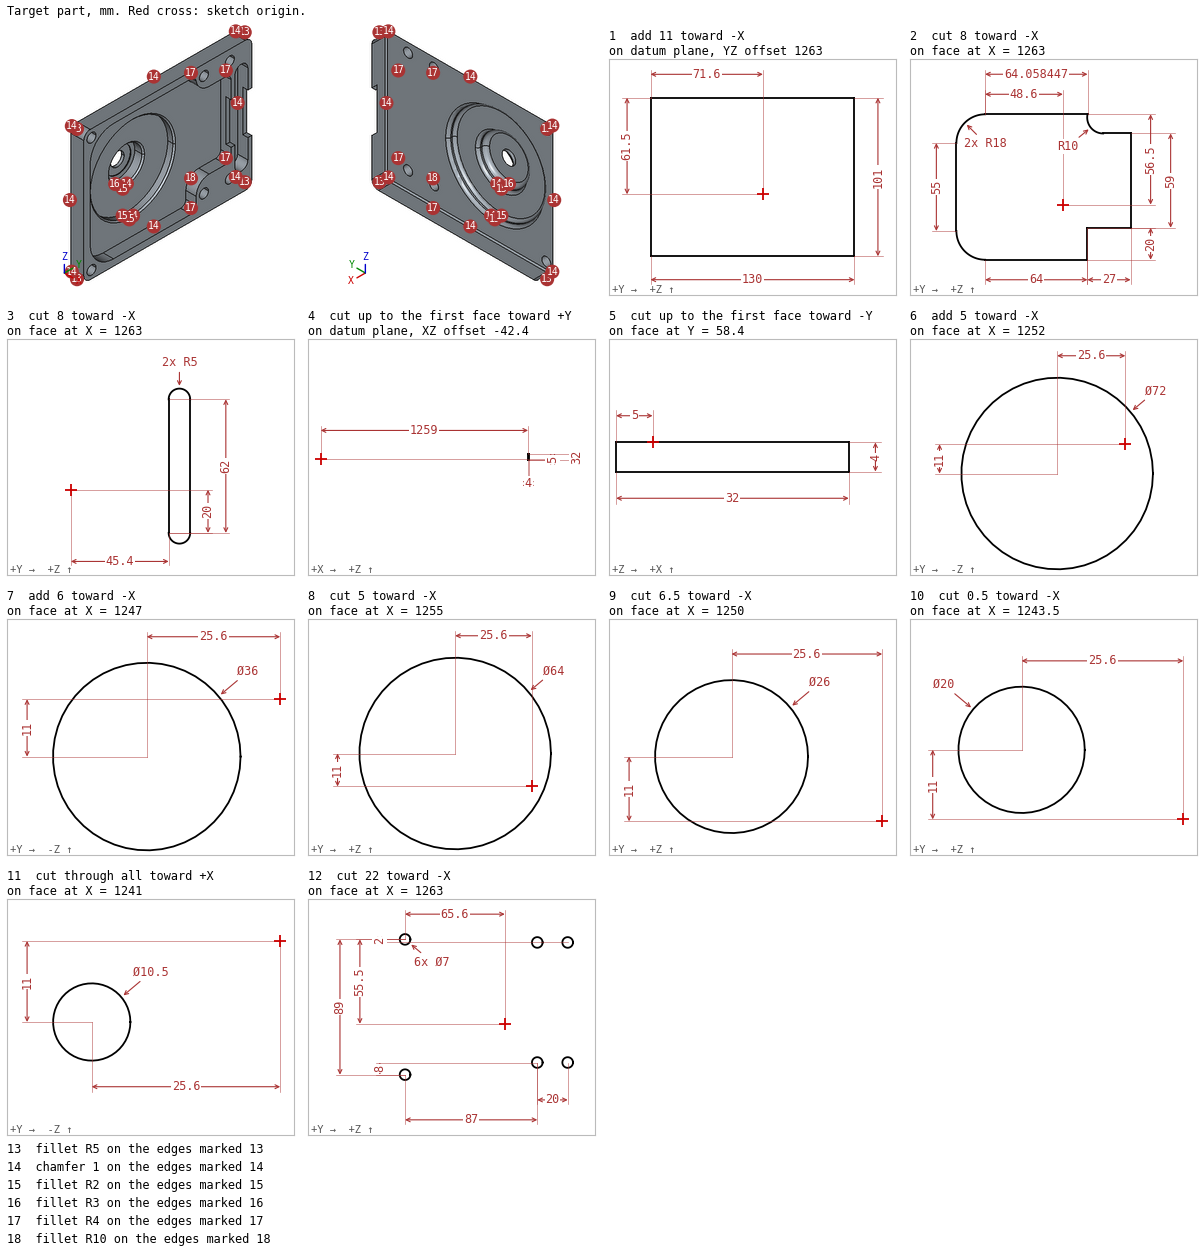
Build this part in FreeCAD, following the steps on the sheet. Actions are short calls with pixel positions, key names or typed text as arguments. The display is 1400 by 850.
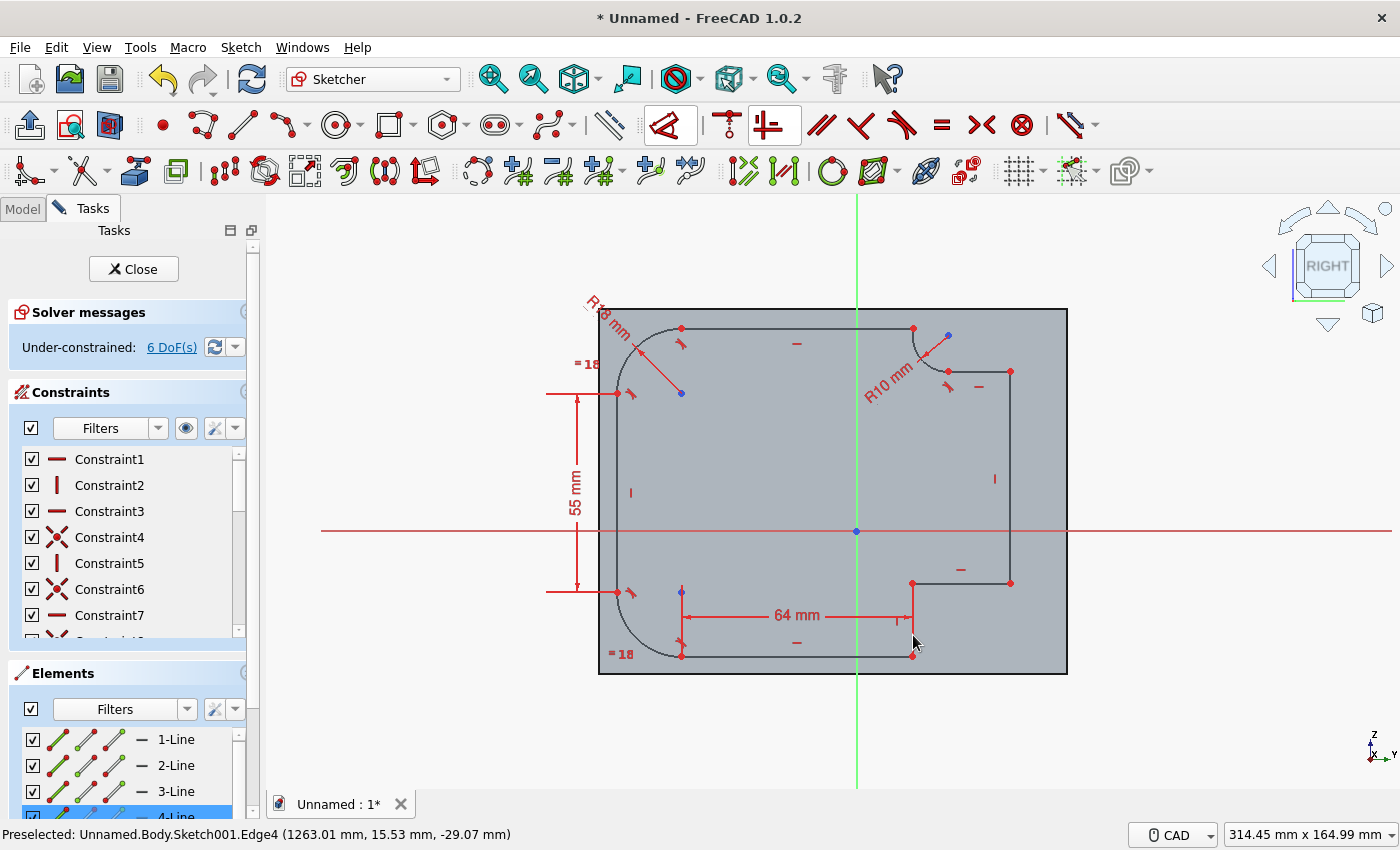
key(i)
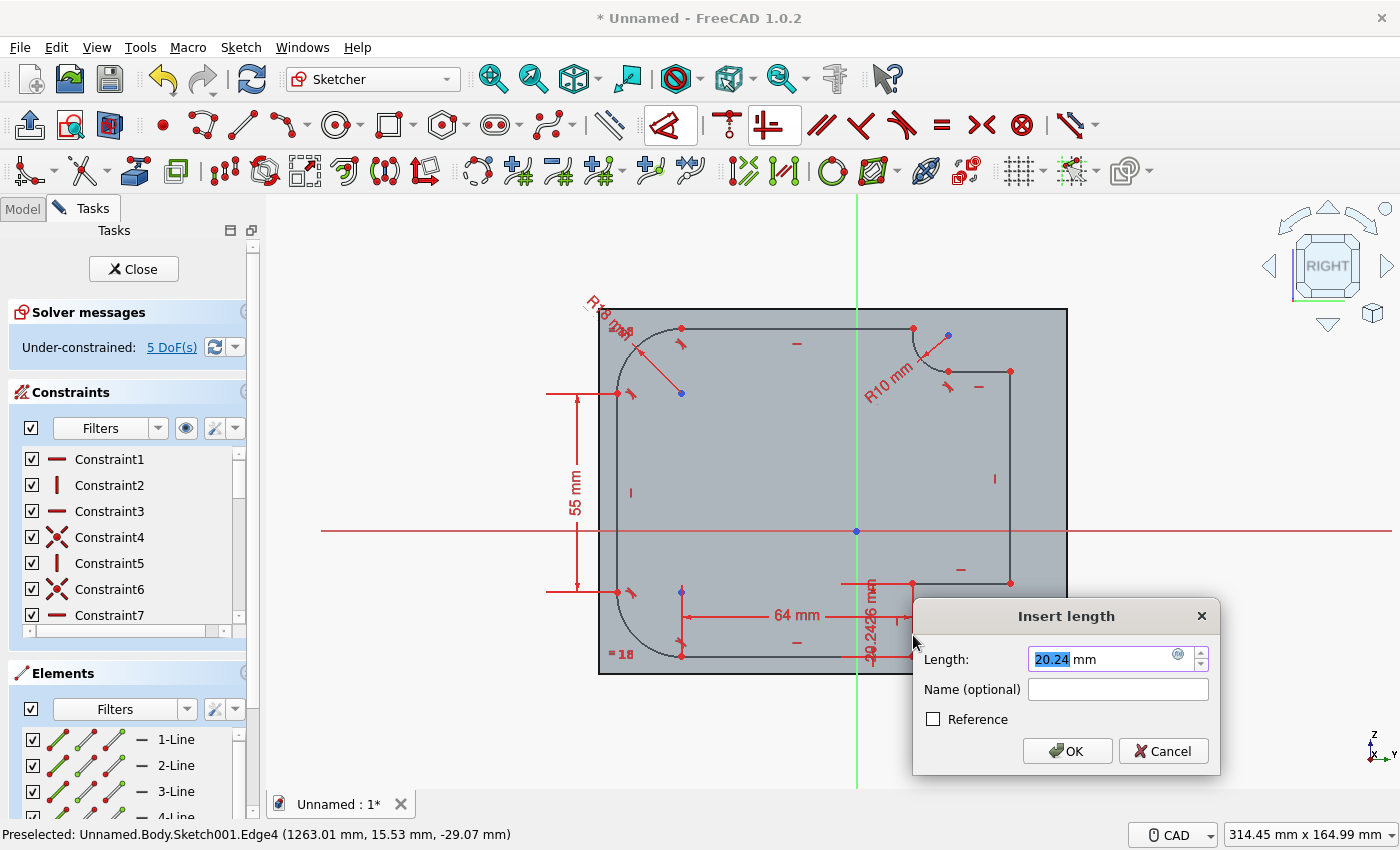
text(20)
key(Return)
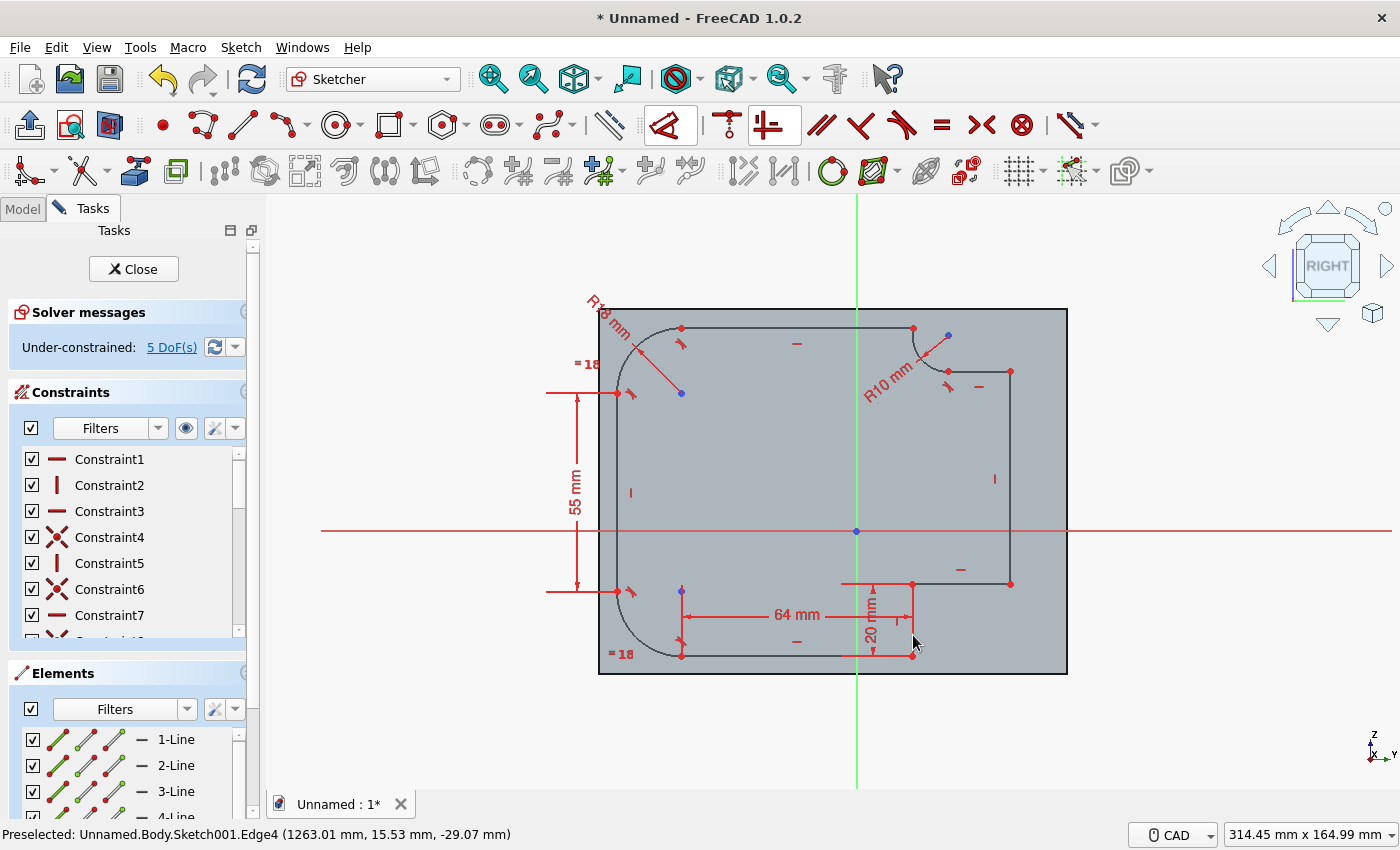
click(942, 584)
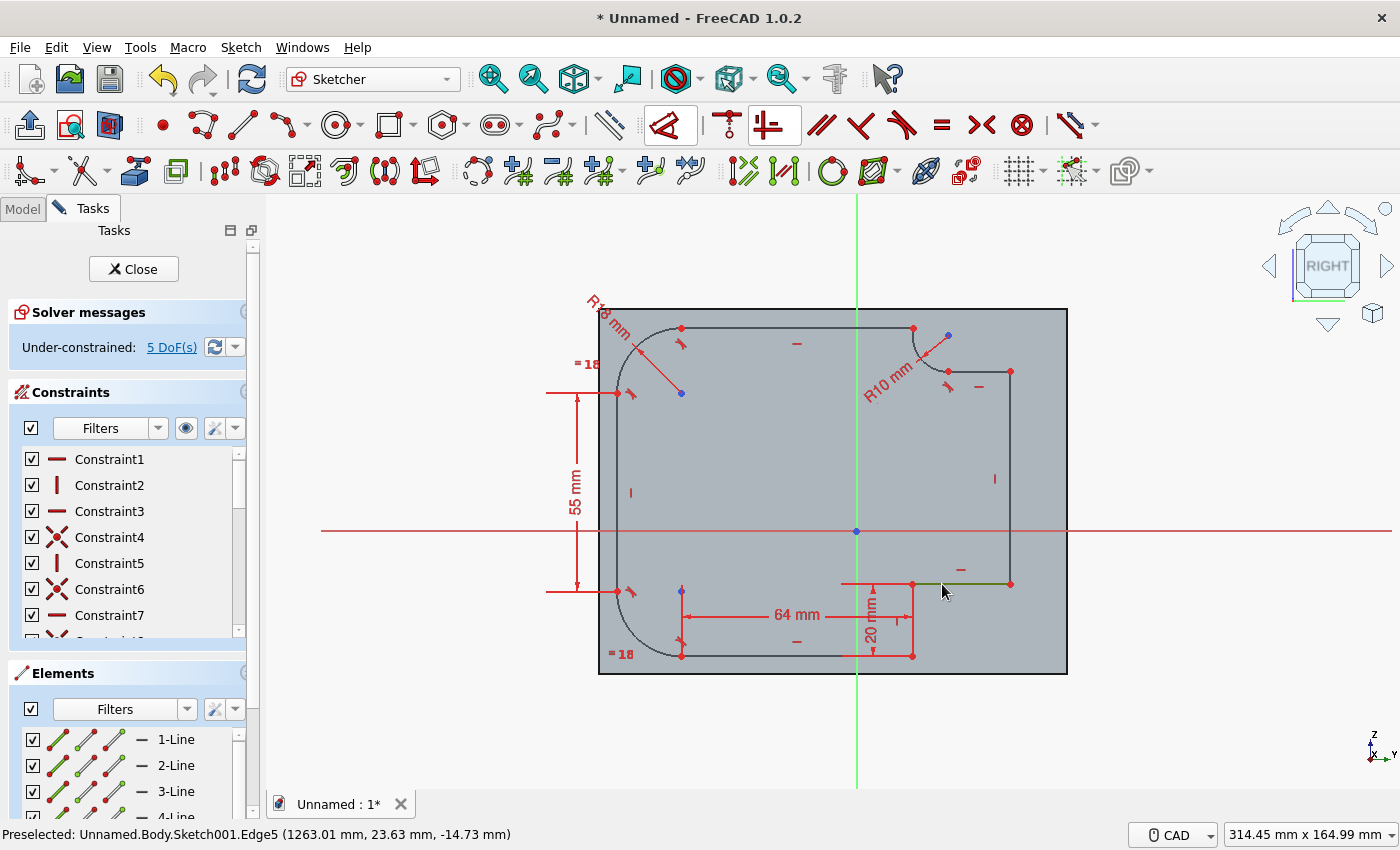
key(l)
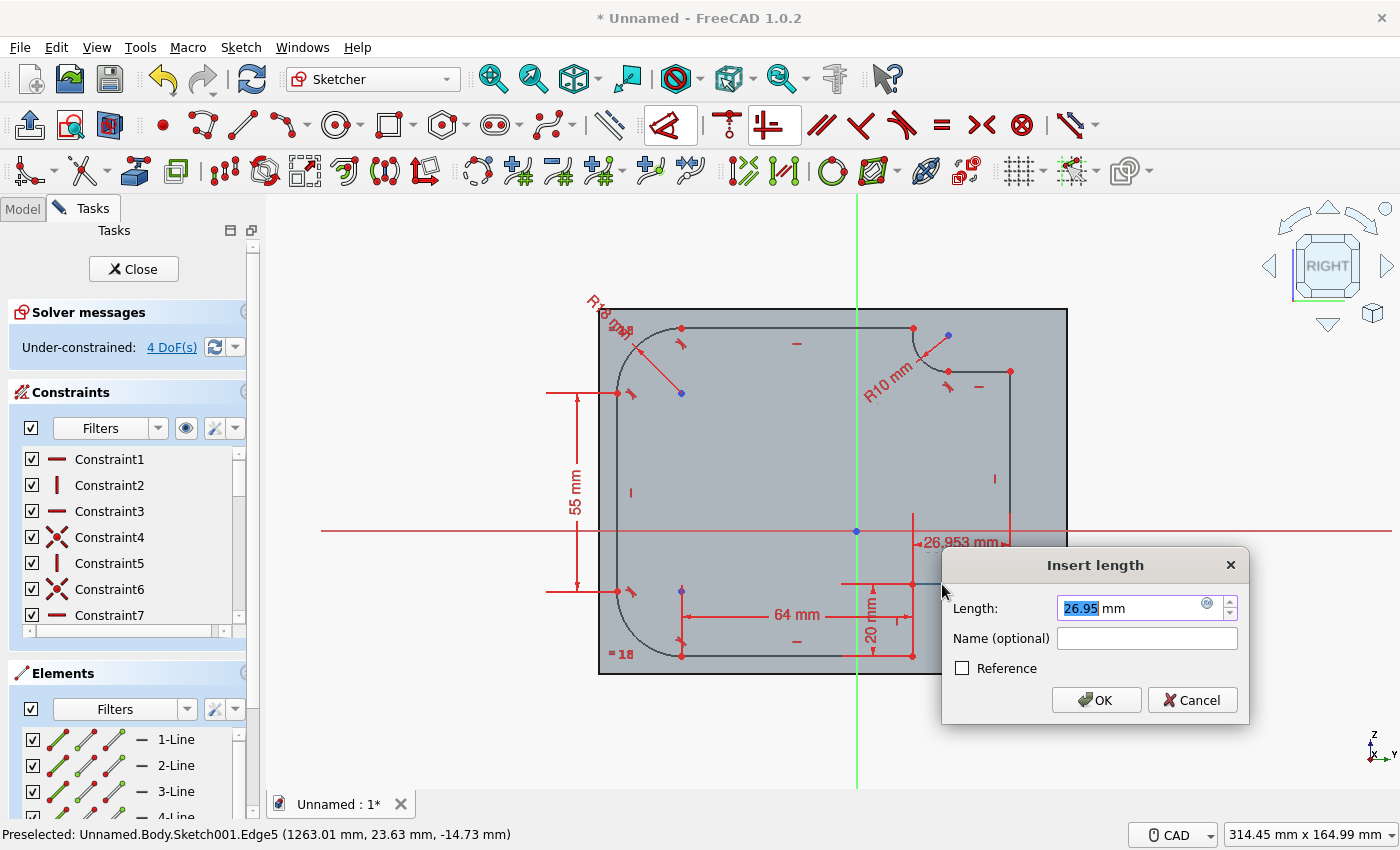
text(27)
key(Return)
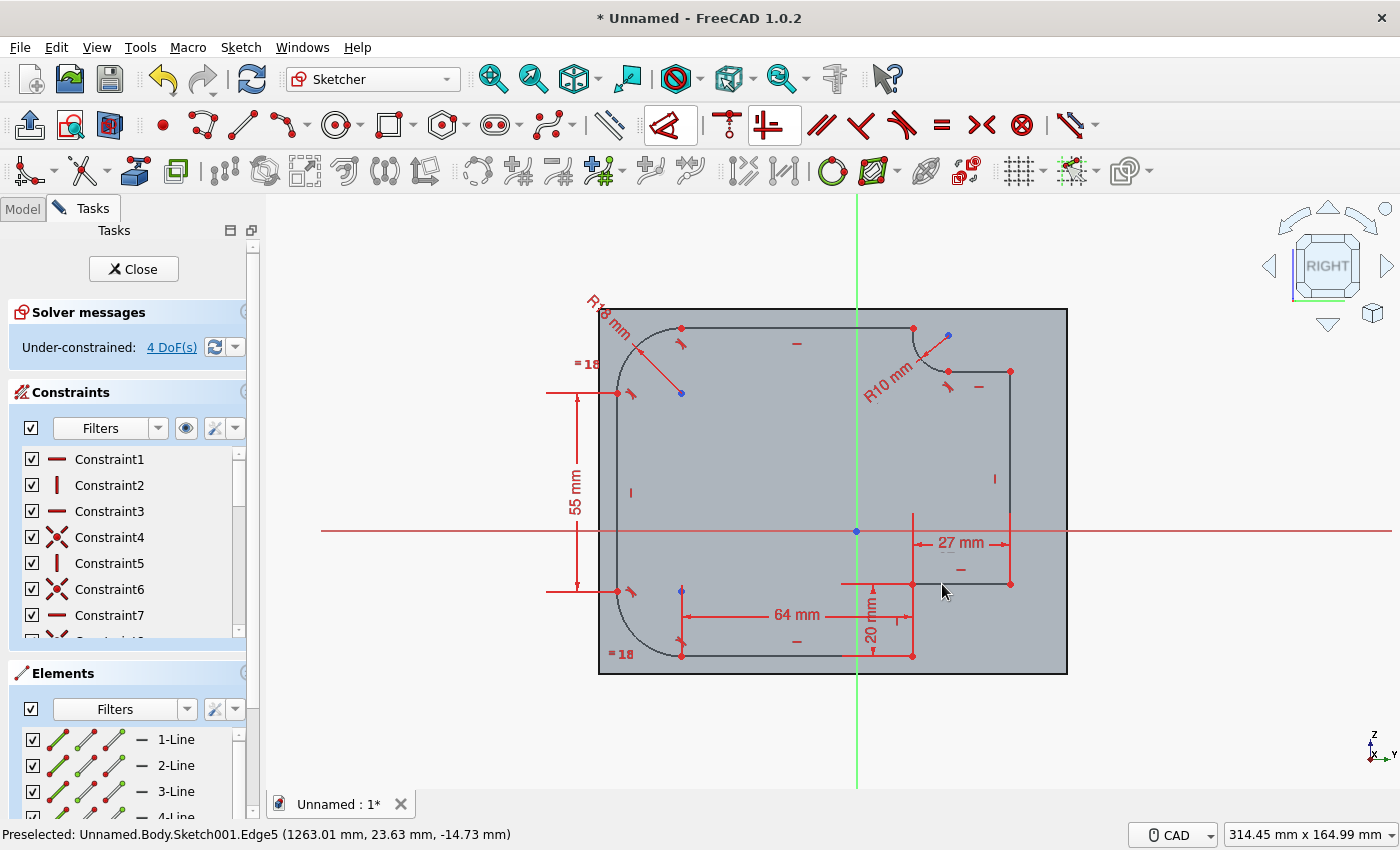
scroll(1010, 521, up, 2)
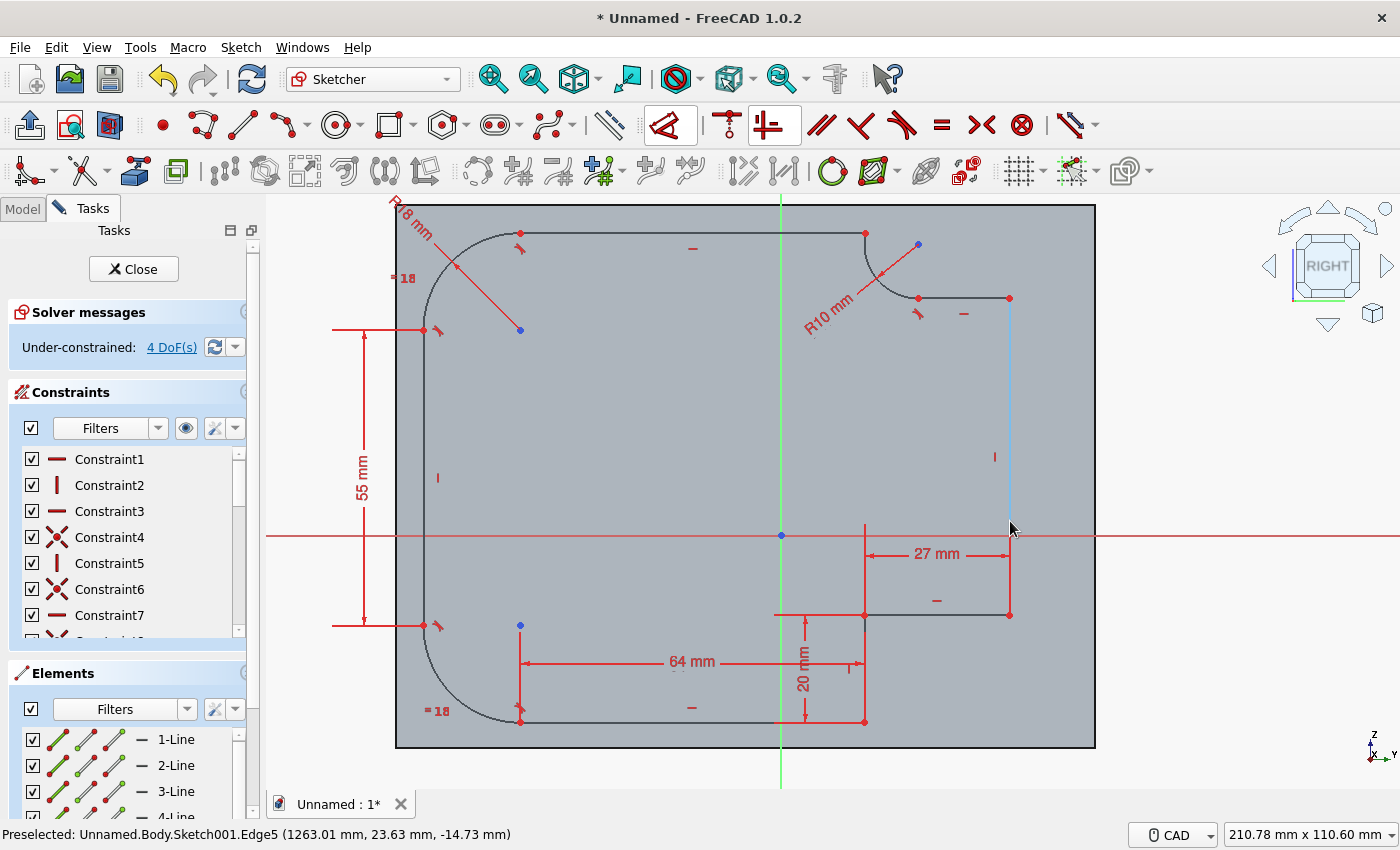
click(1010, 520)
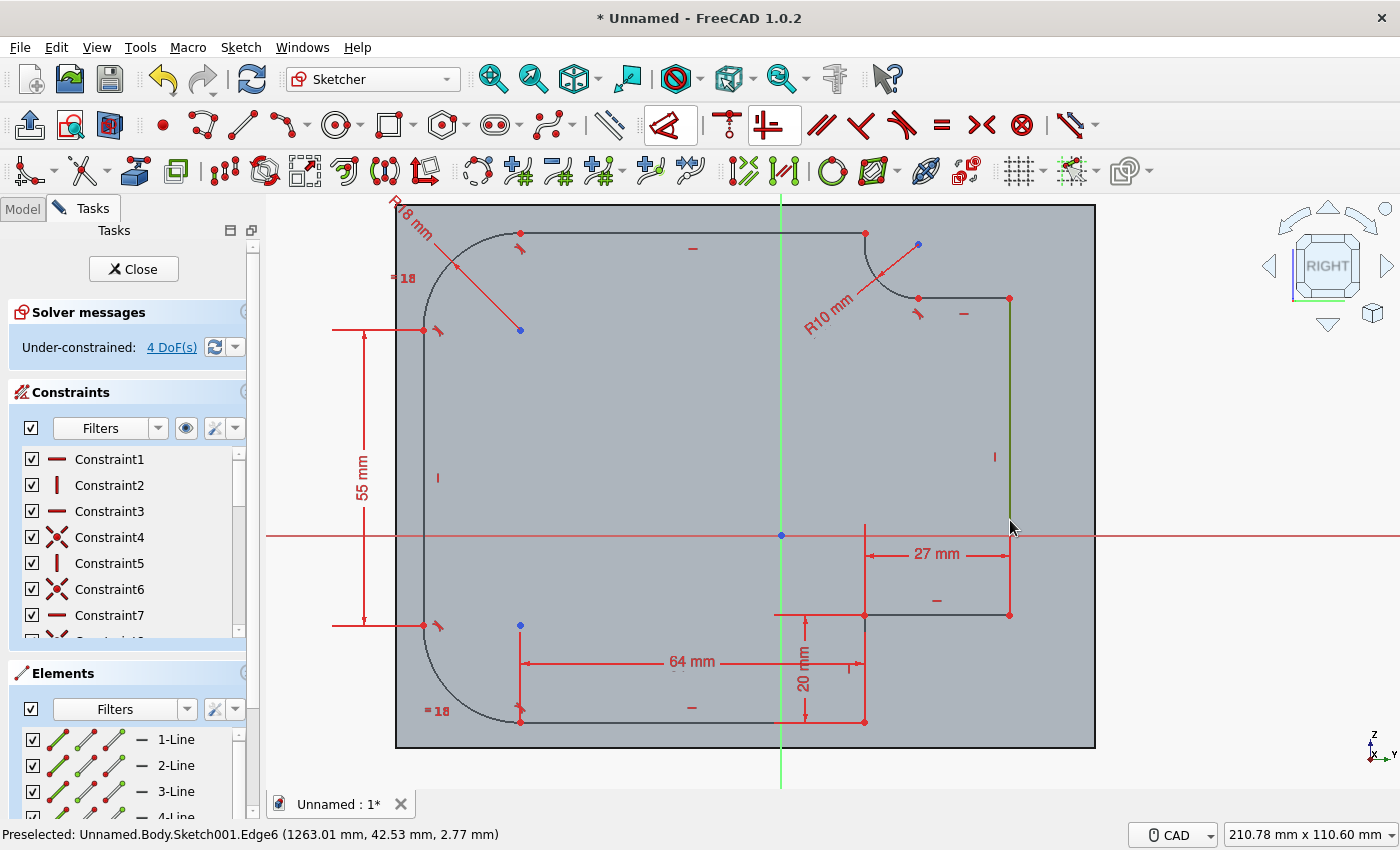
click(692, 126)